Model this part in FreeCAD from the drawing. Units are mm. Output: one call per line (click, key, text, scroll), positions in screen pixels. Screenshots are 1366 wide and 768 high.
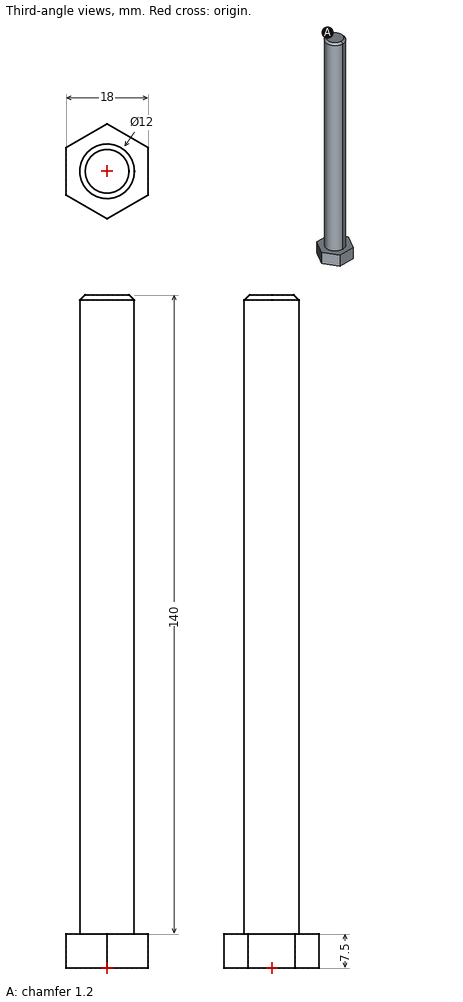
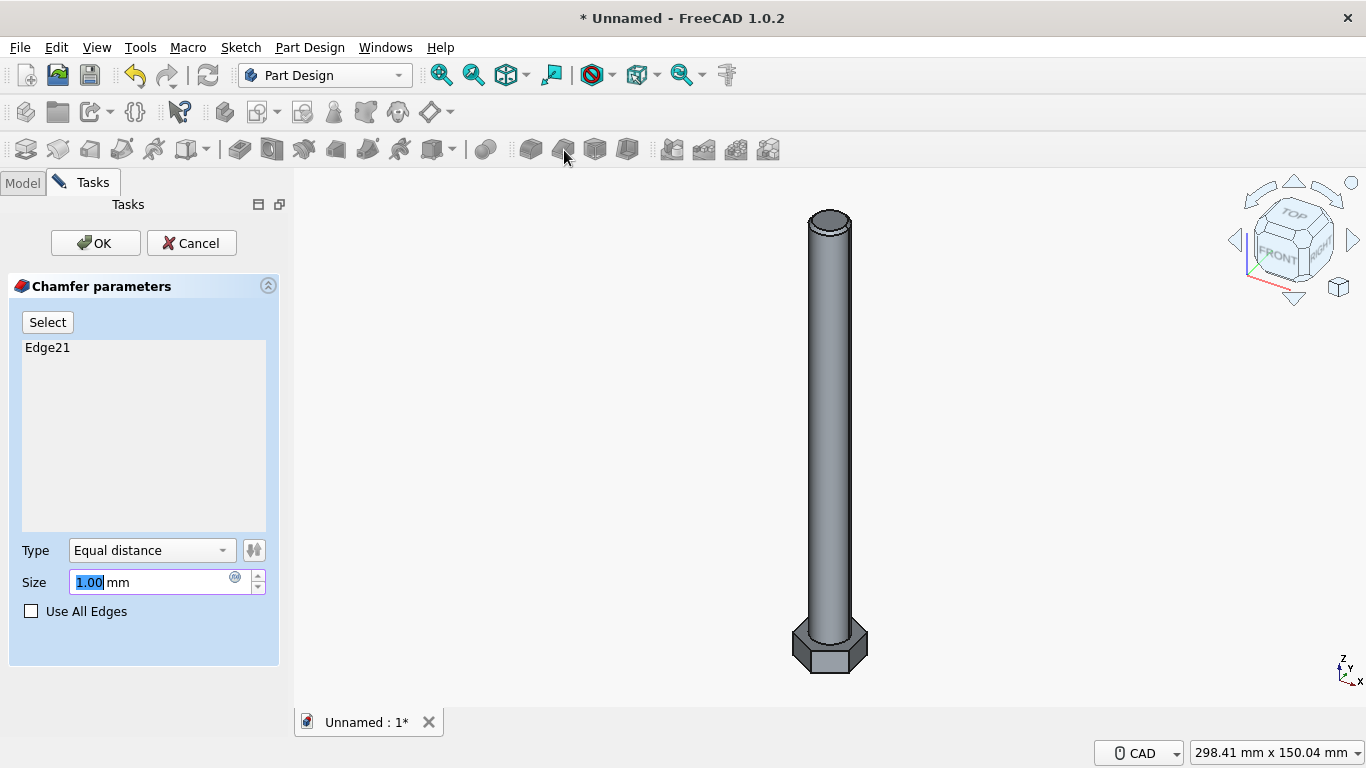
text(1.2)
key(Tab)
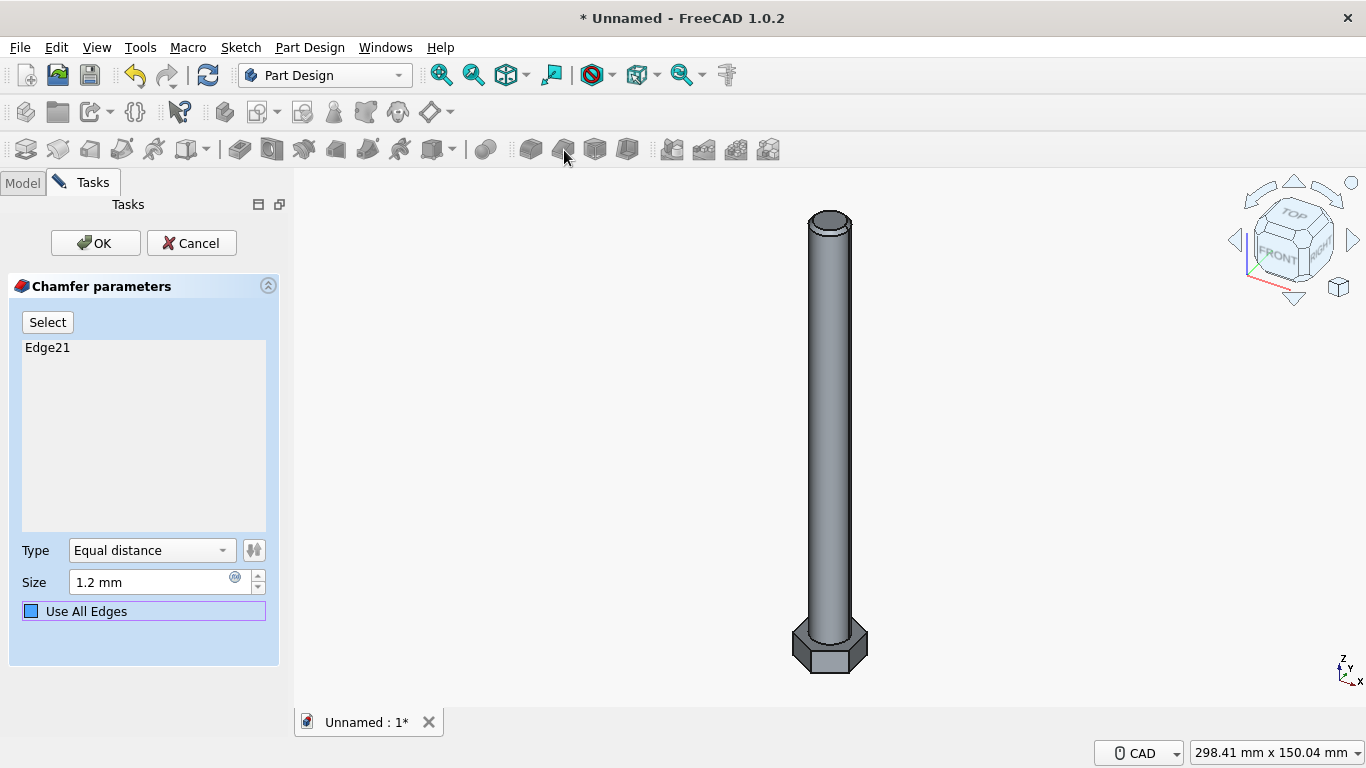
click(96, 243)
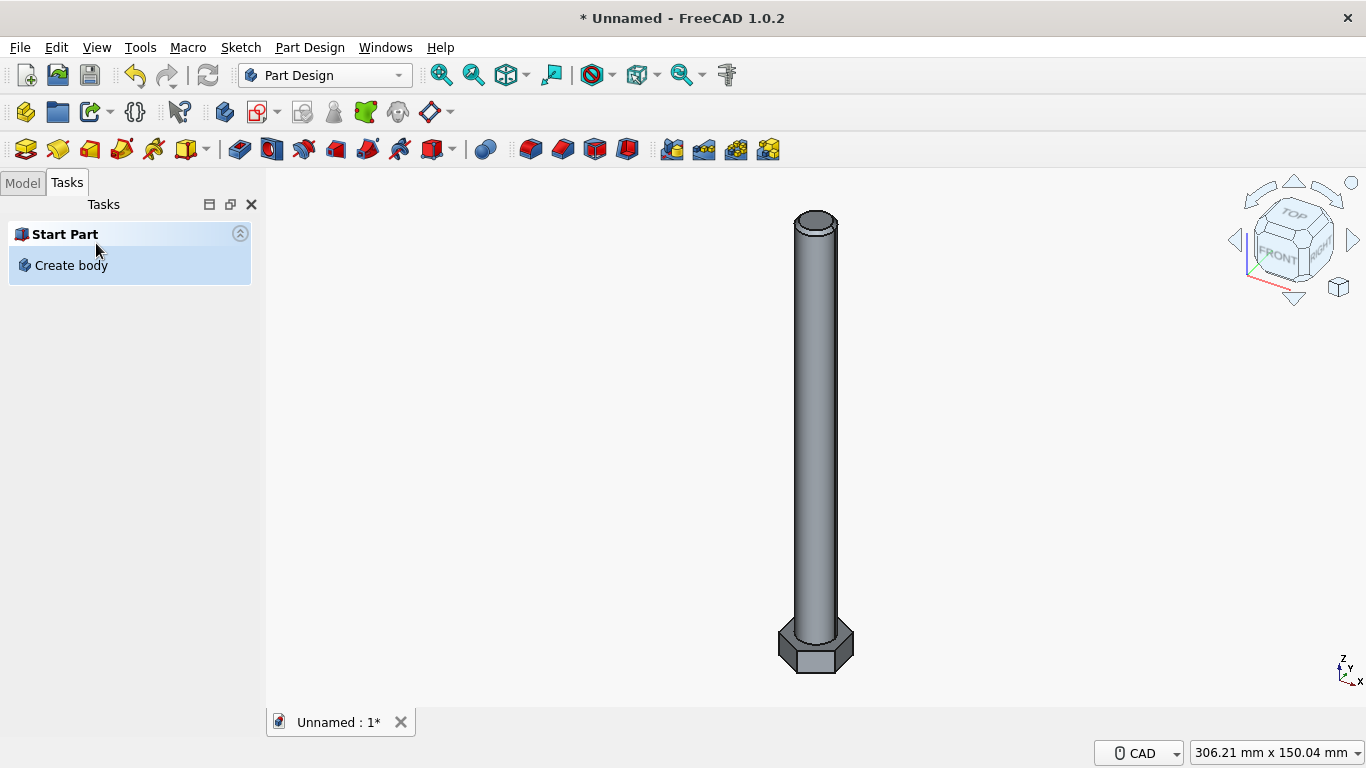
key(0)